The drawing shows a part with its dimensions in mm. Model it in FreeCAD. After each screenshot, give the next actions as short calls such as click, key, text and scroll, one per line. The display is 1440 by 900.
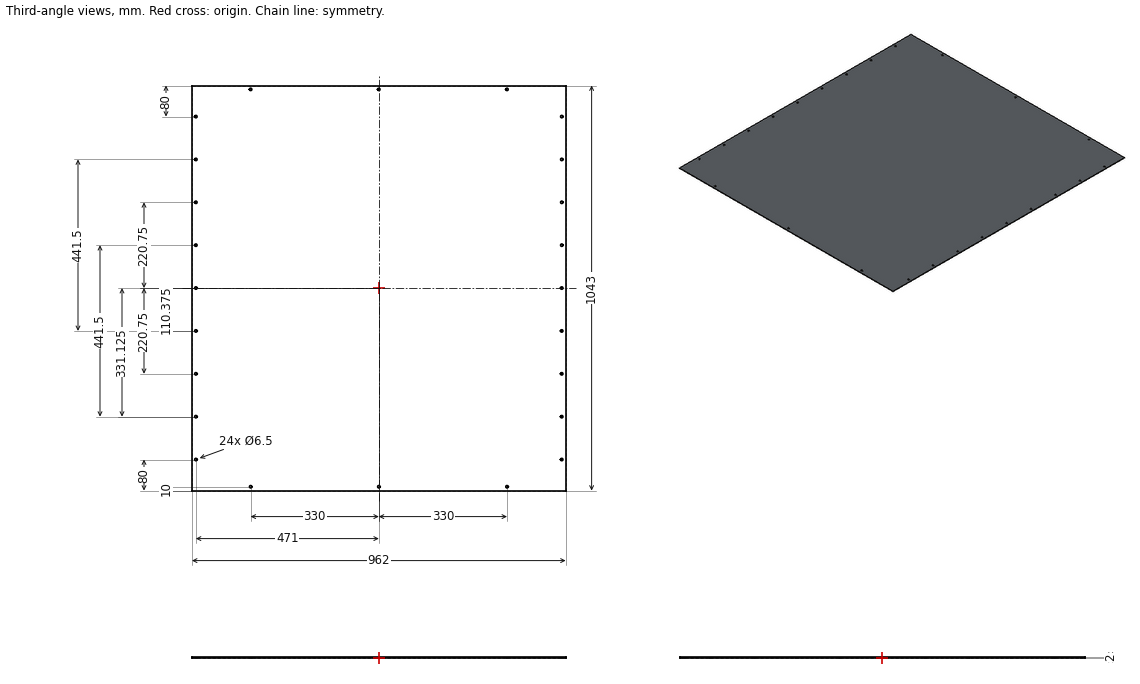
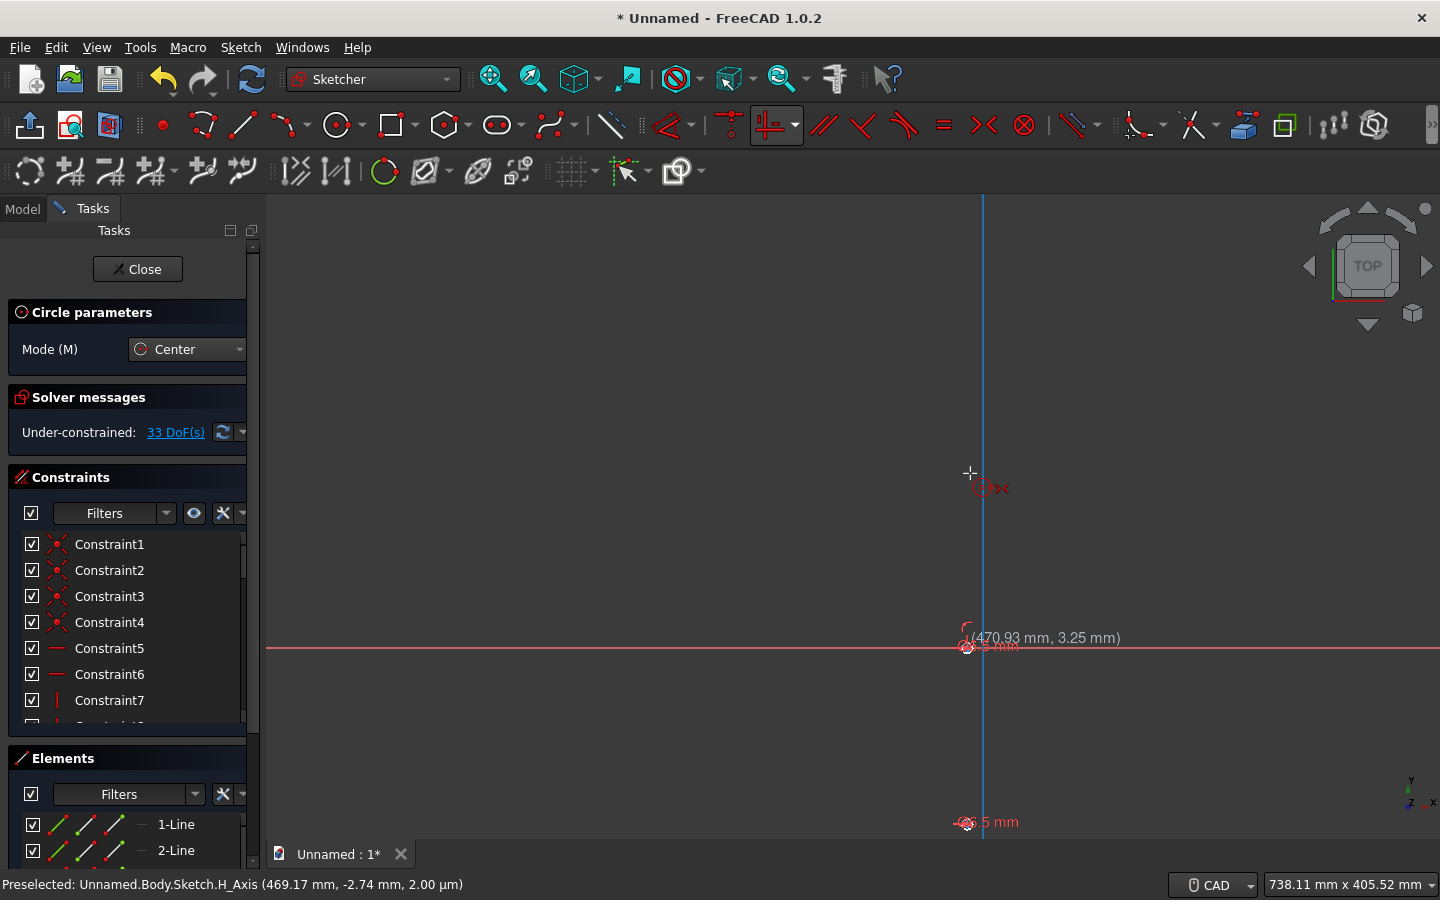
click(967, 473)
move(964, 469)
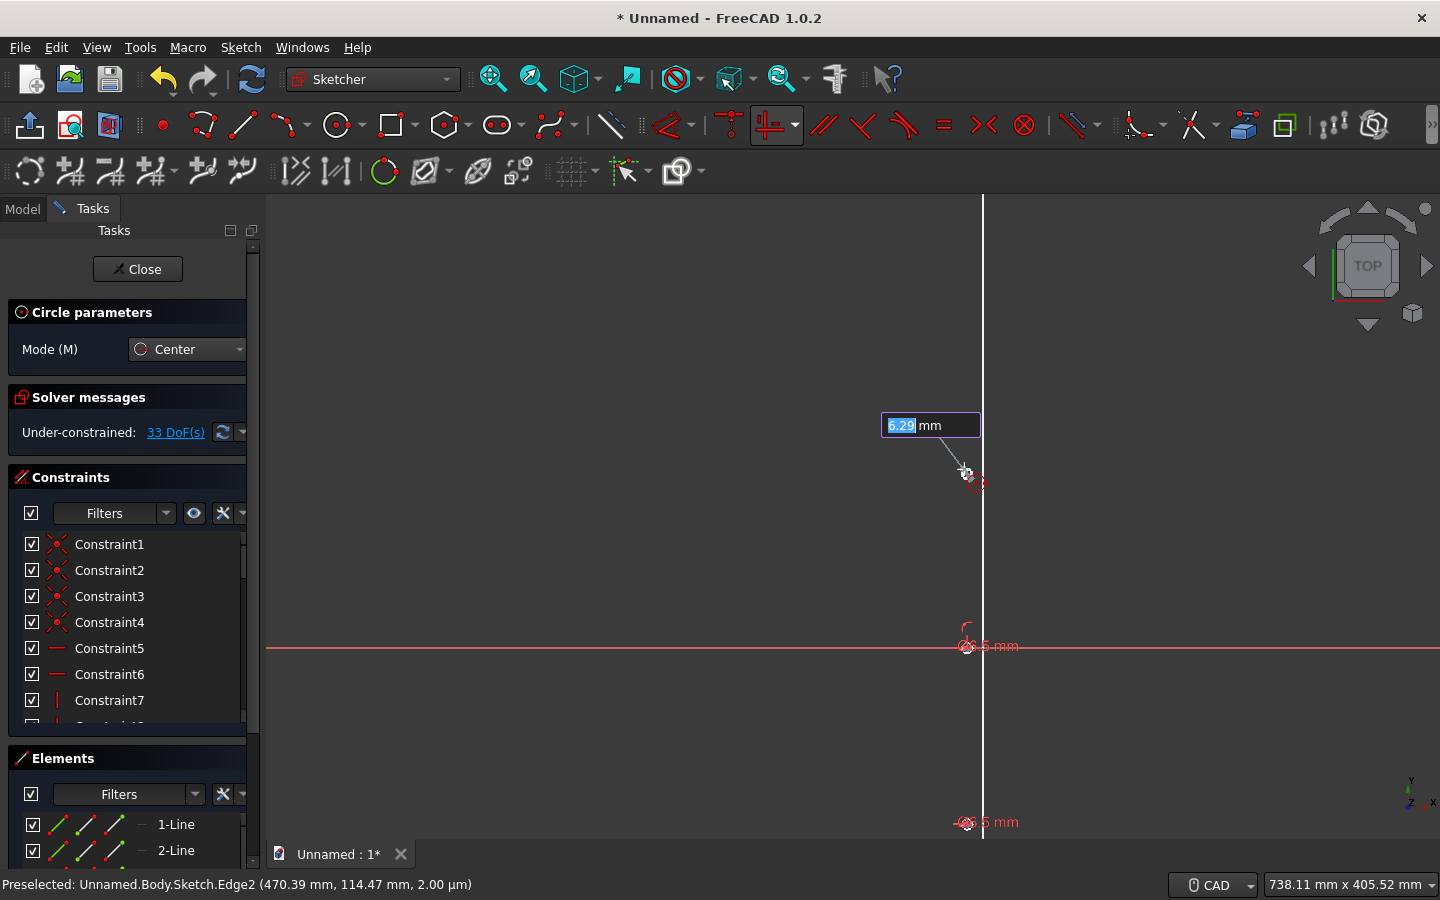
text(6.5)
key(Return)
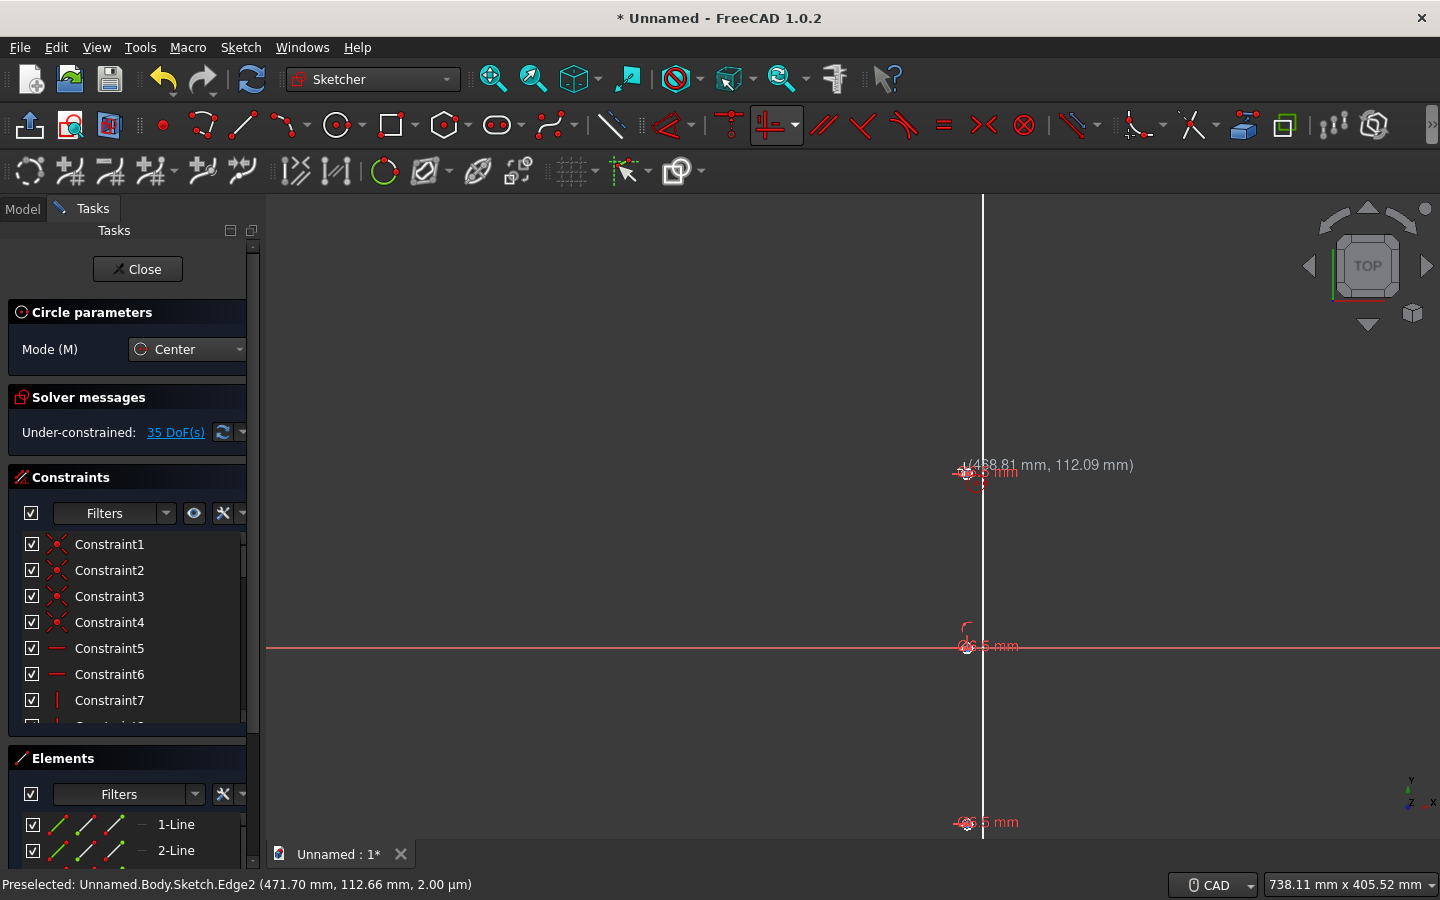
scroll(967, 297, up, 8)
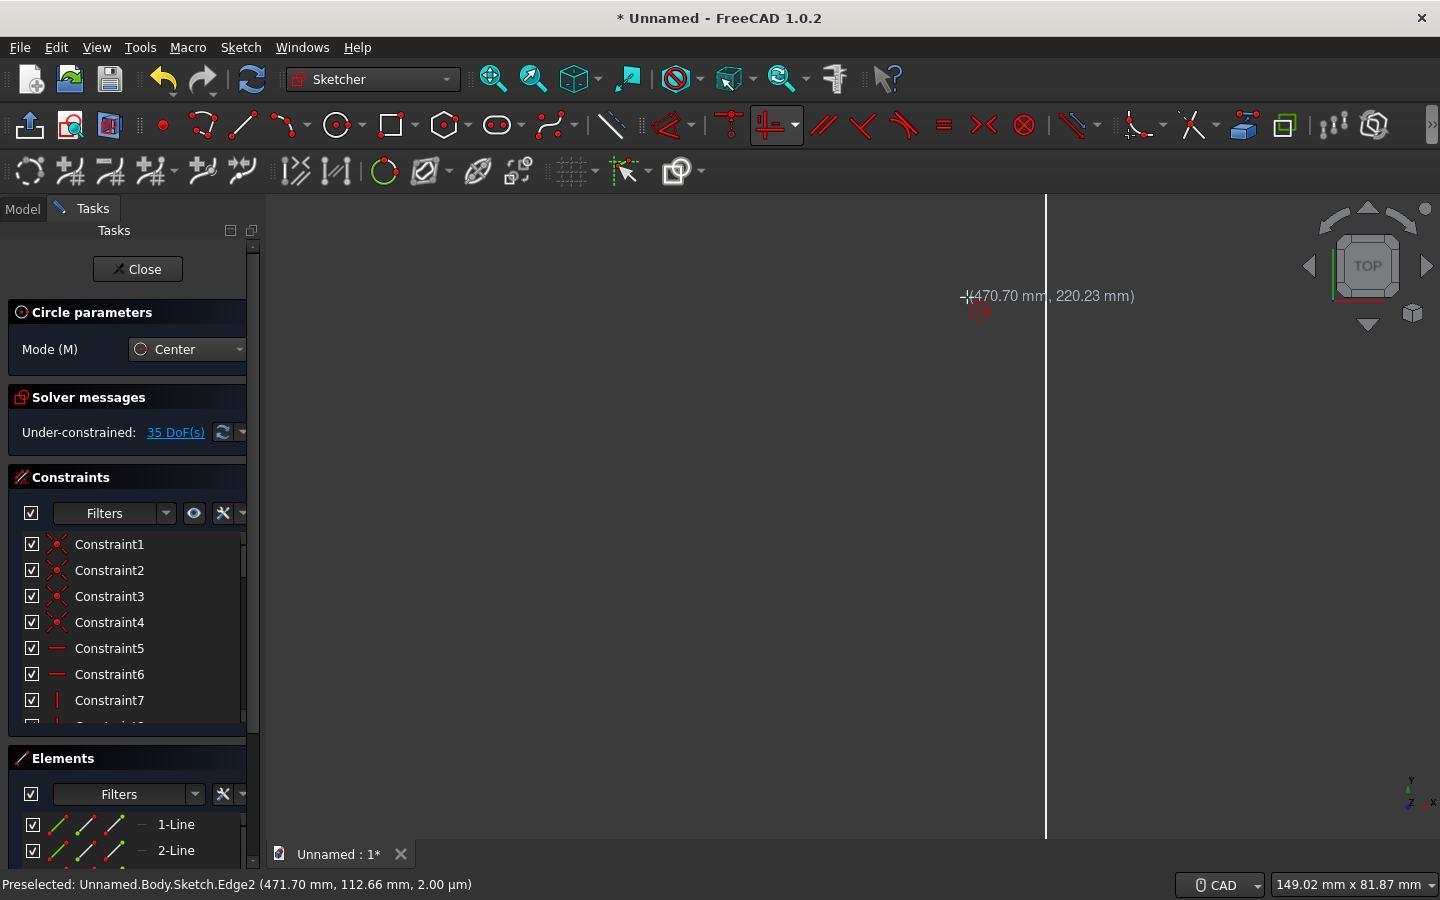
scroll(969, 437, down, 15)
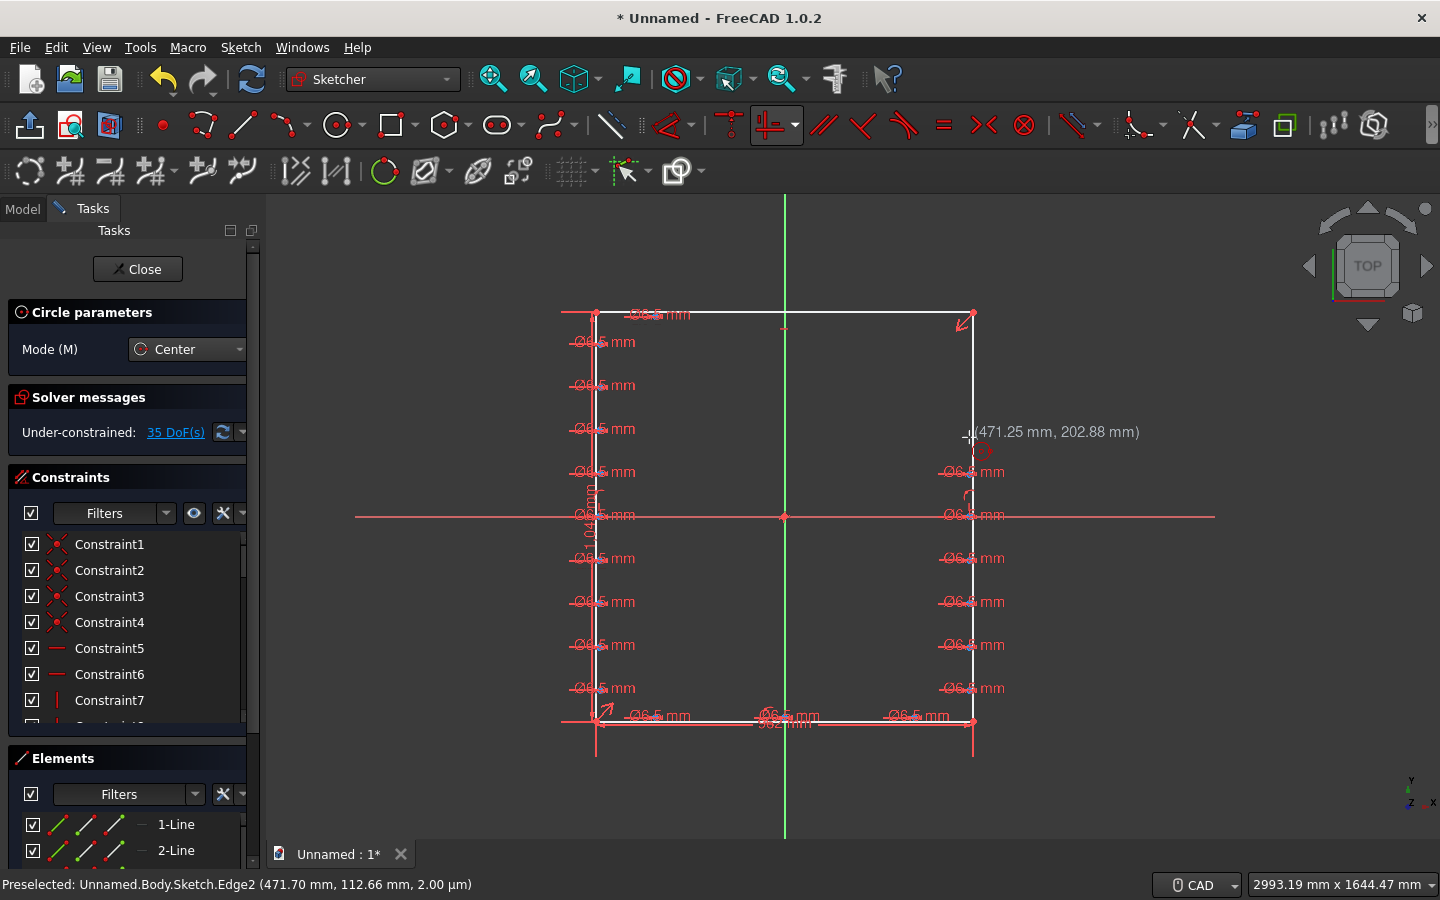
scroll(969, 430, up, 7)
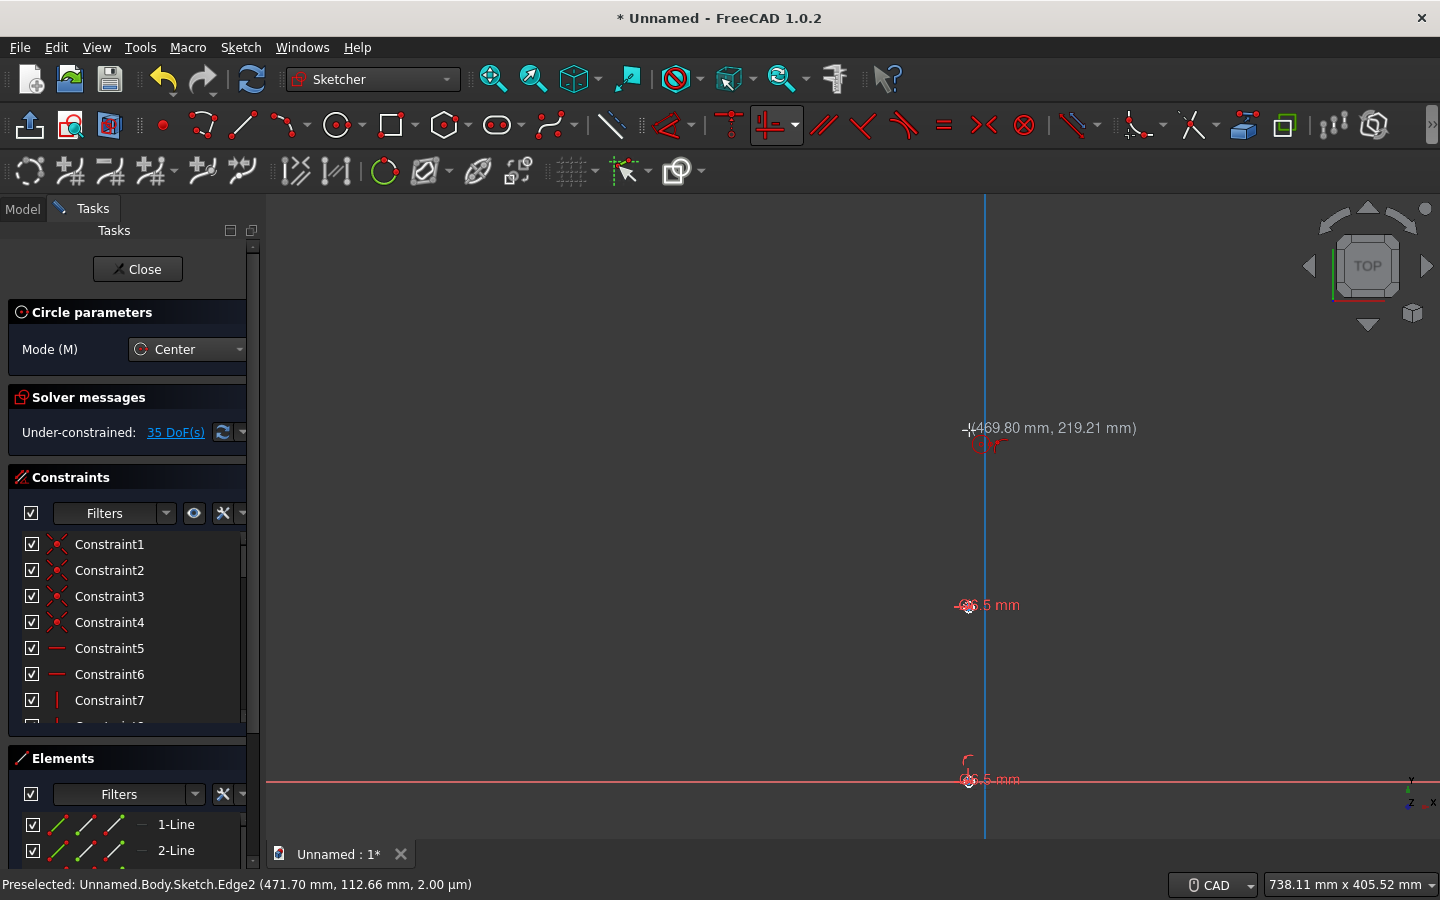
click(969, 430)
move(965, 427)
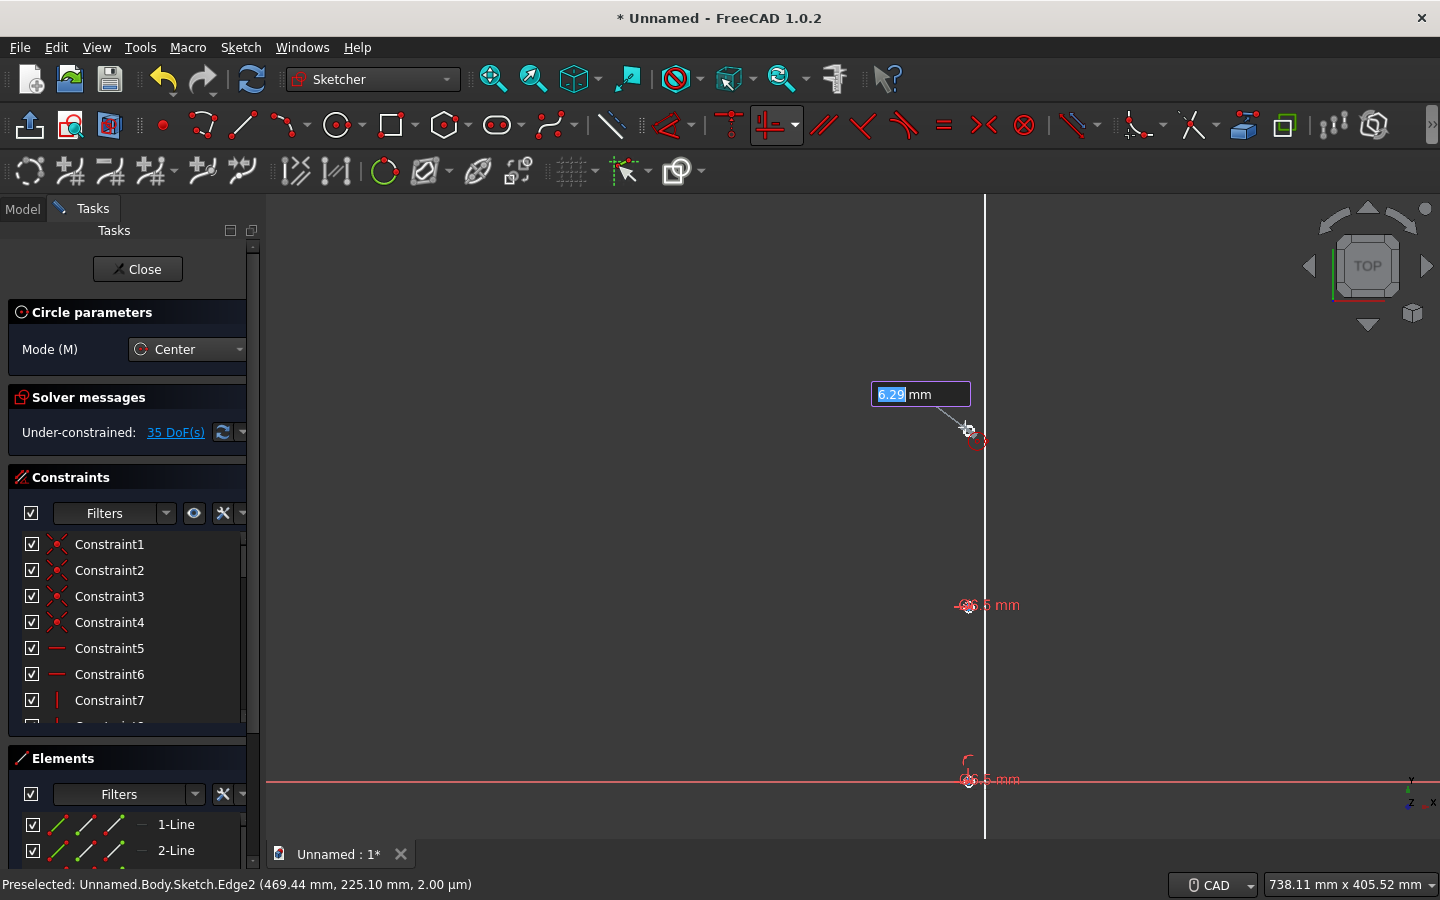
text(6.5)
key(Return)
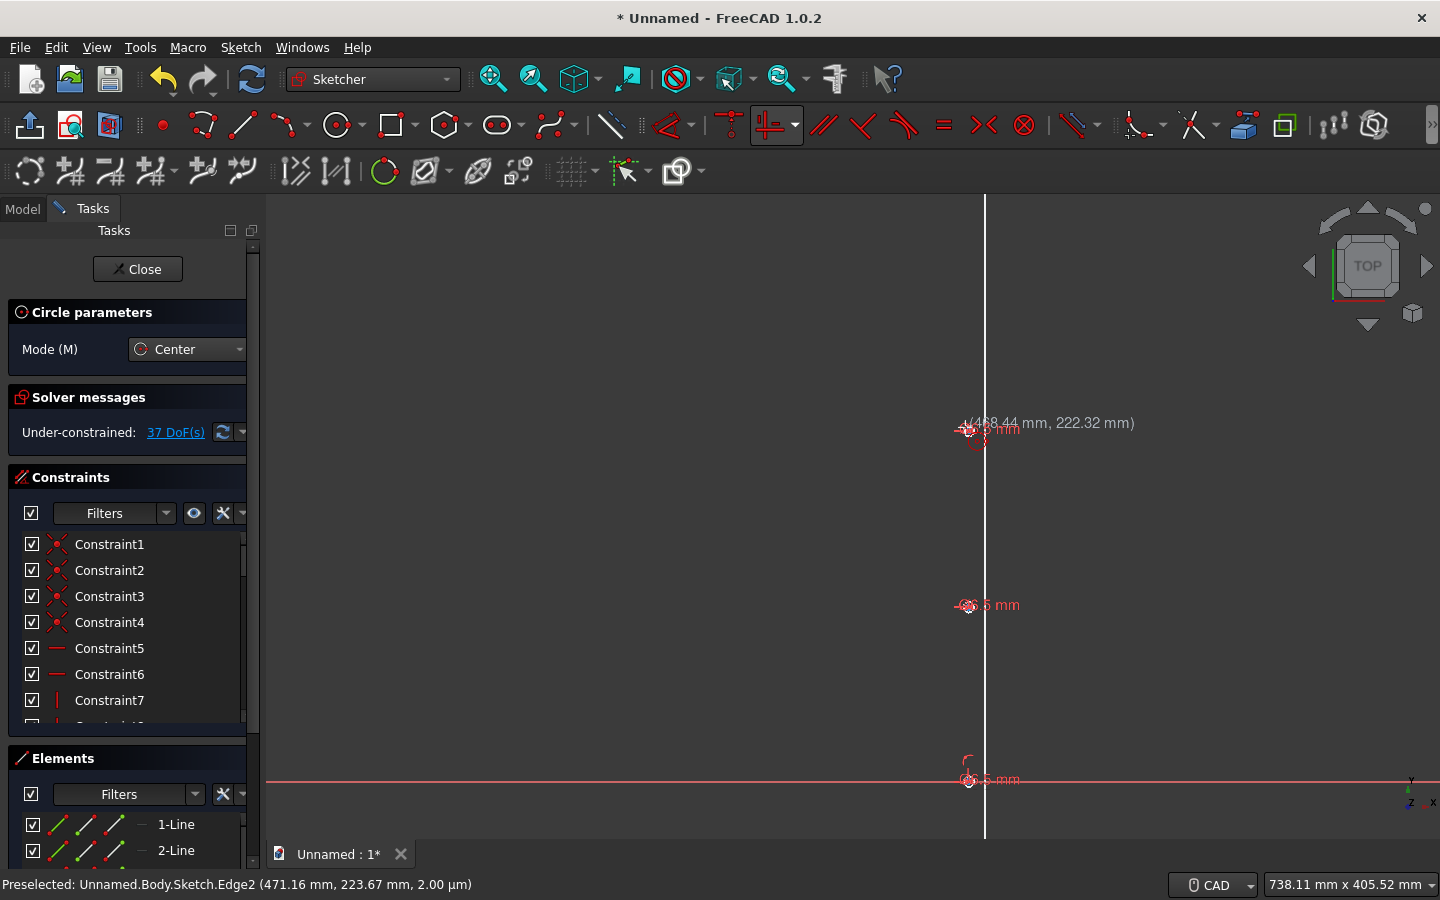
scroll(969, 430, down, 7)